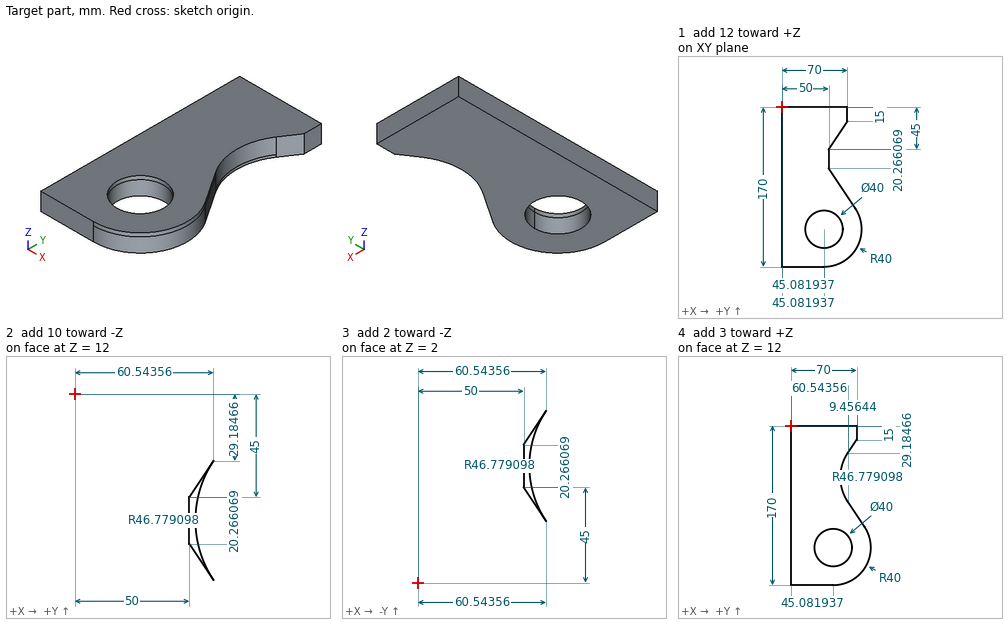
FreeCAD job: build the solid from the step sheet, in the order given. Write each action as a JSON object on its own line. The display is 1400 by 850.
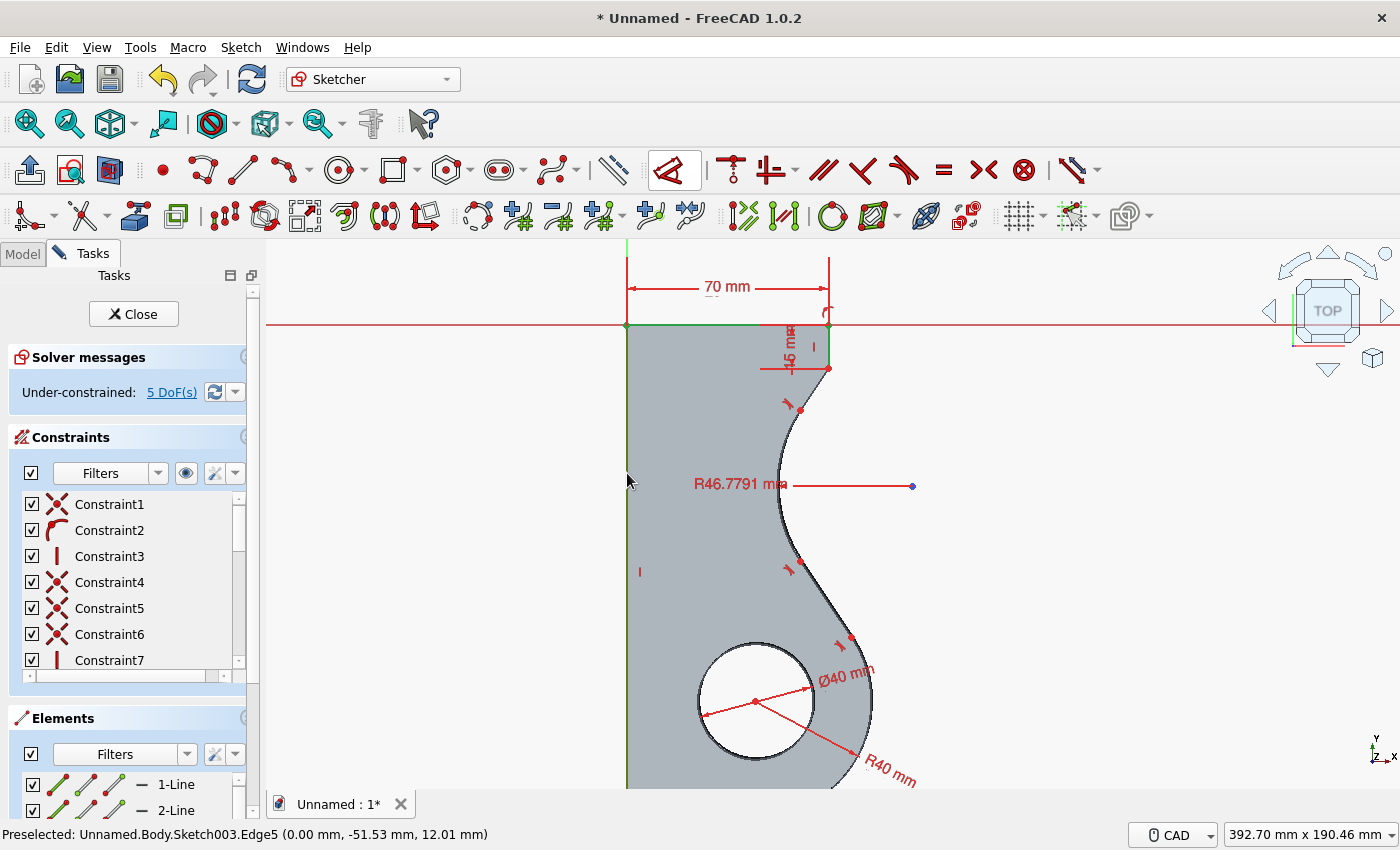
{"action": "key", "text": "i"}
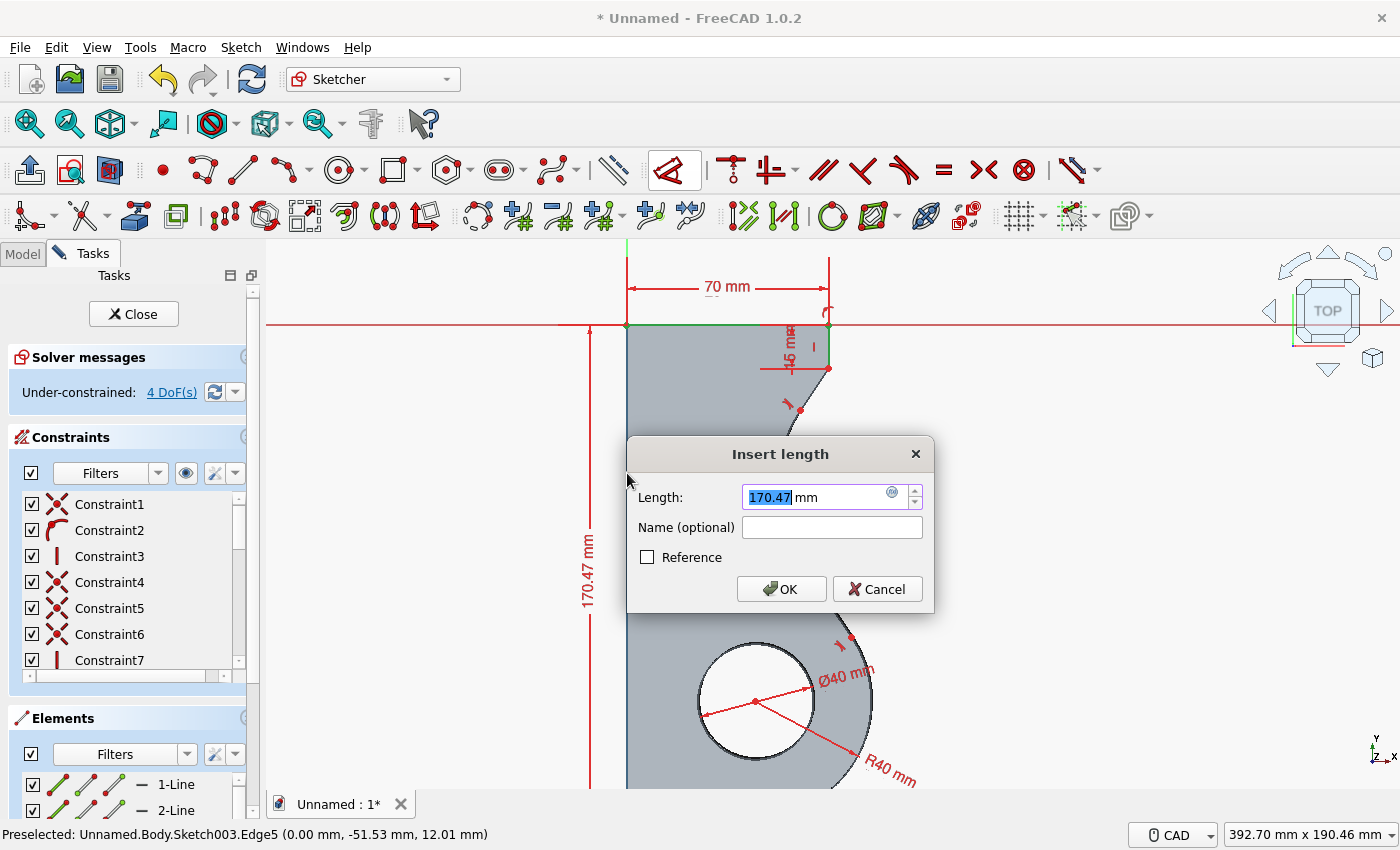
{"action": "type", "text": "170"}
{"action": "key", "text": "Return"}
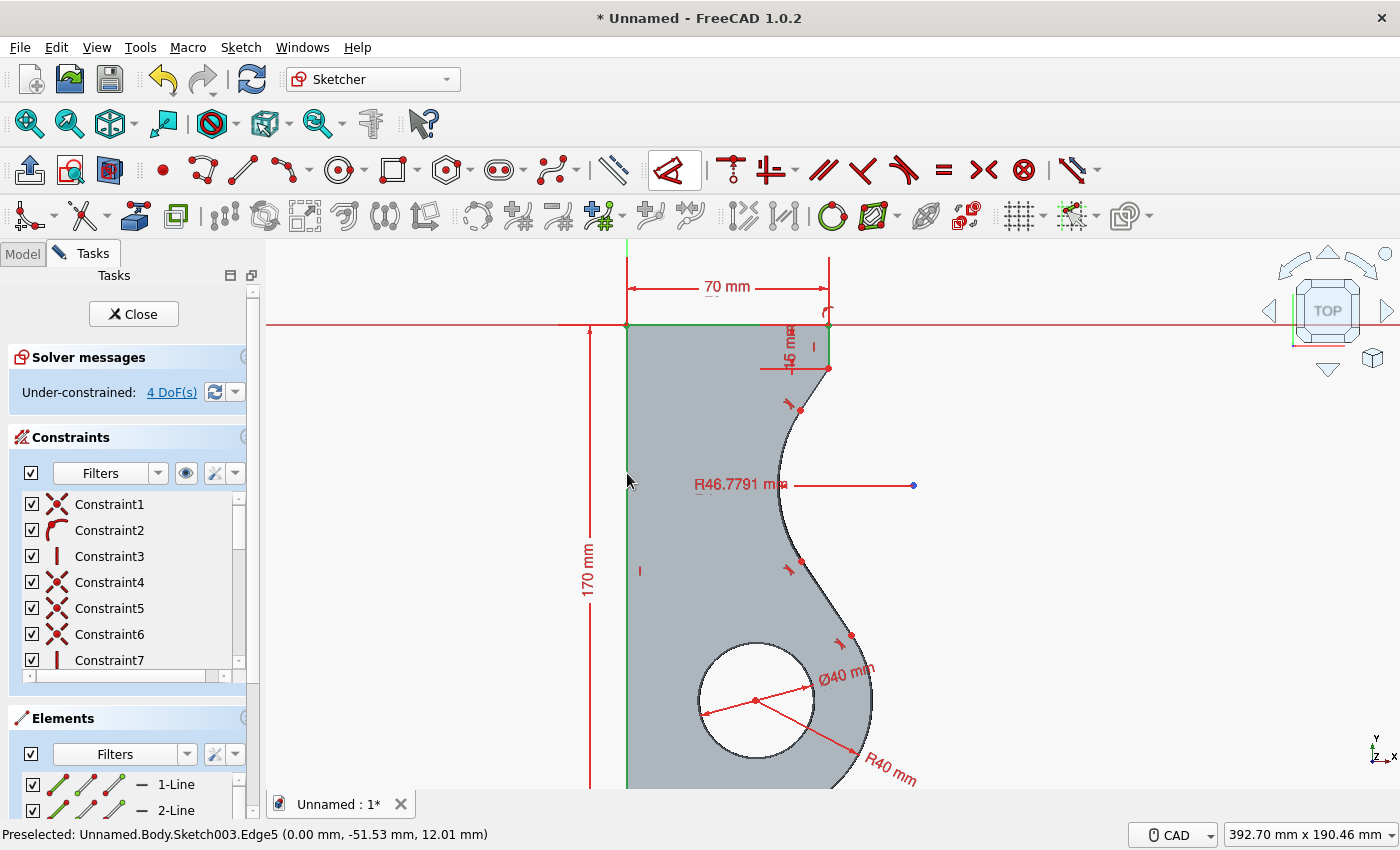
{"action": "scroll", "coordinate": [809, 398], "scroll_direction": "up", "scroll_amount": 2}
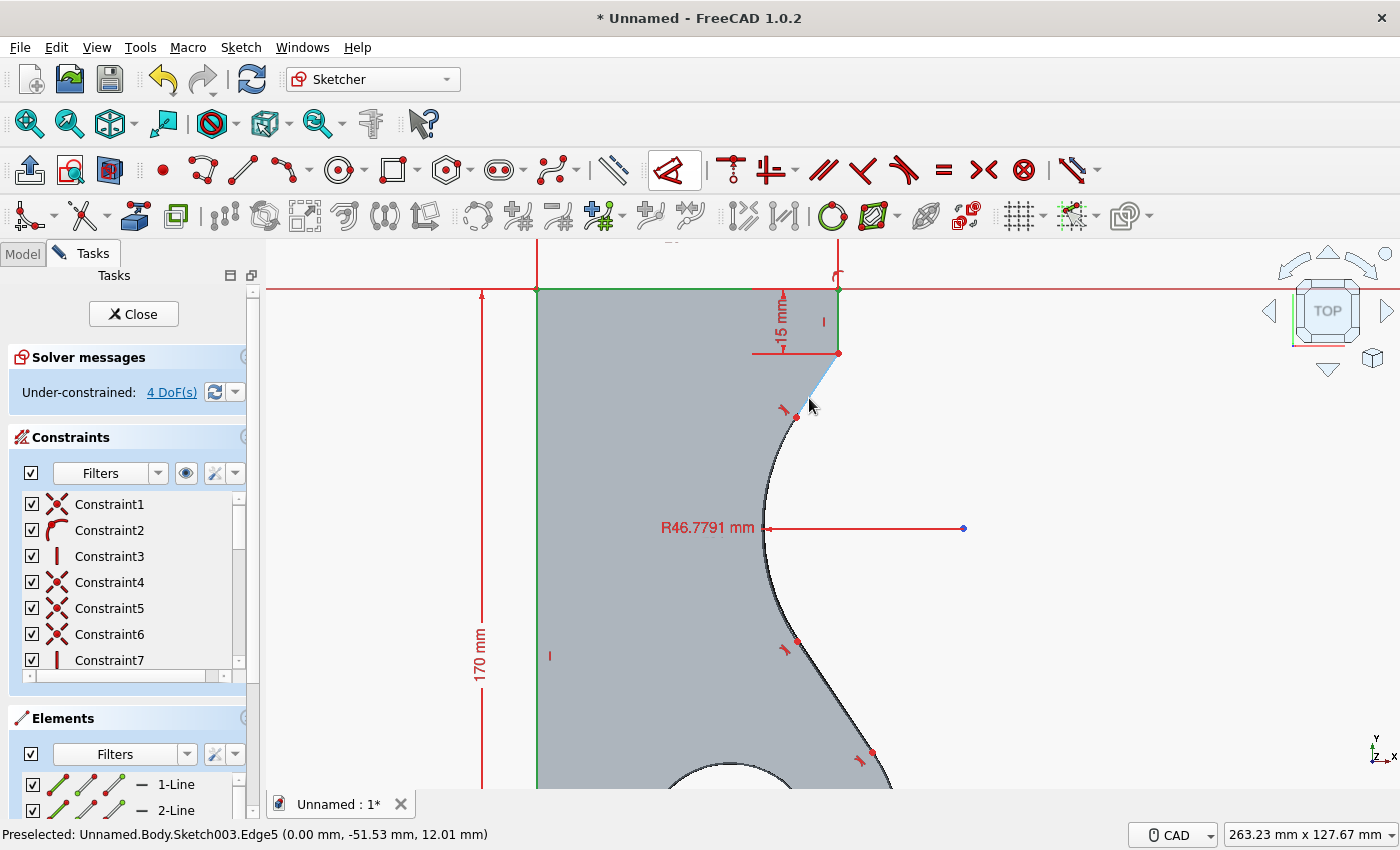
{"action": "left_click", "coordinate": [809, 398]}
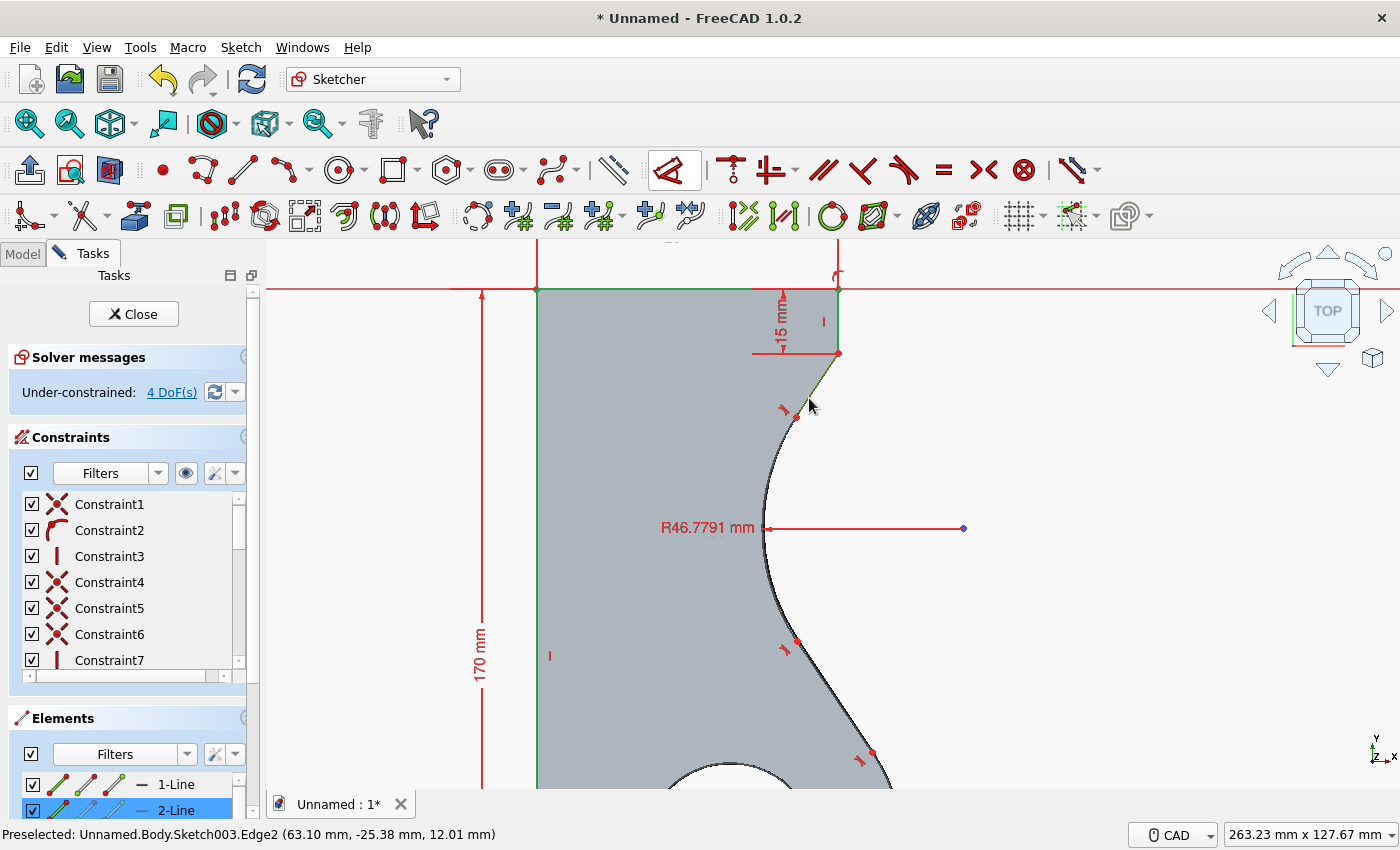
{"action": "key", "text": "l"}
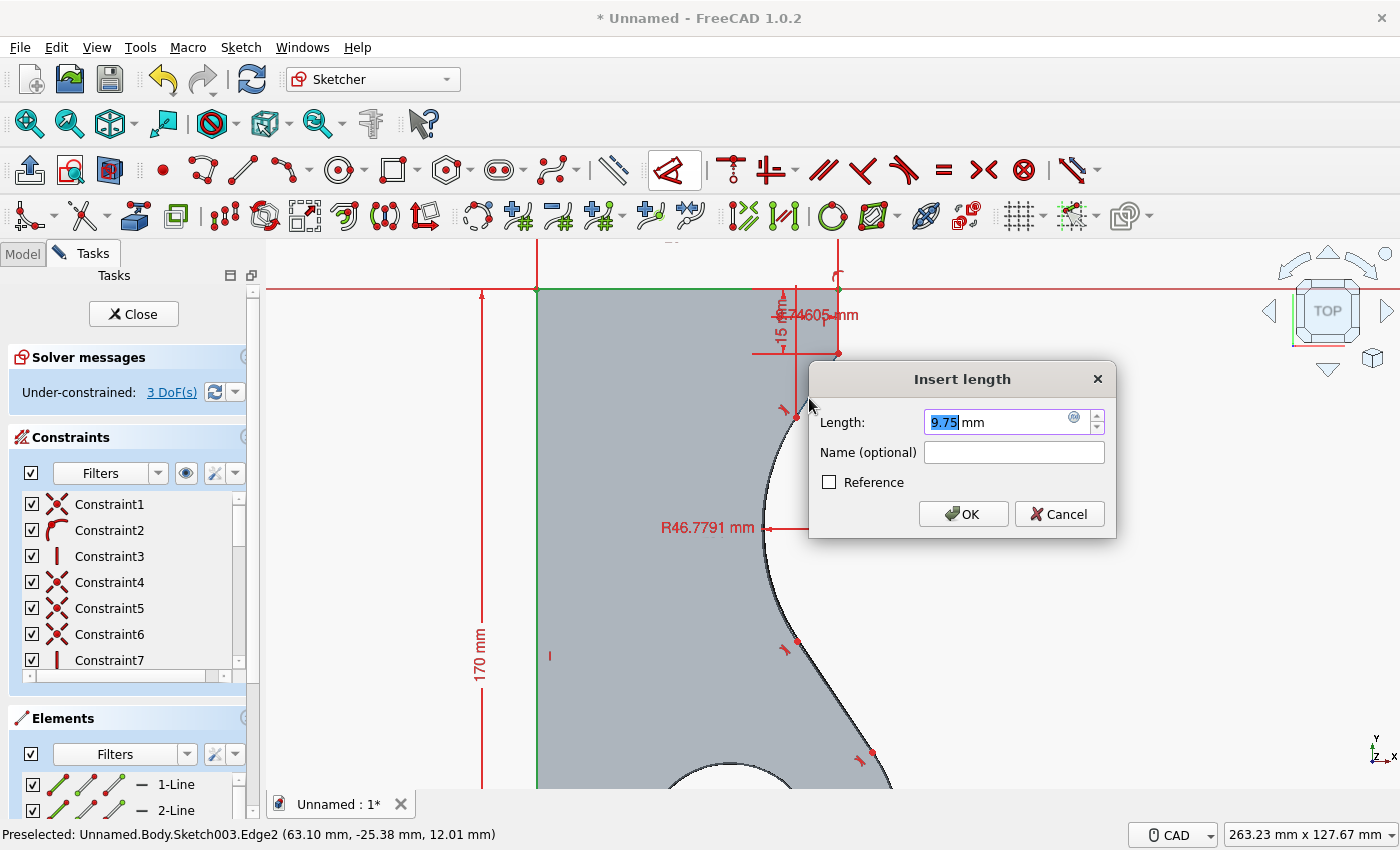
{"action": "type", "text": "9.45644"}
{"action": "key", "text": "Return"}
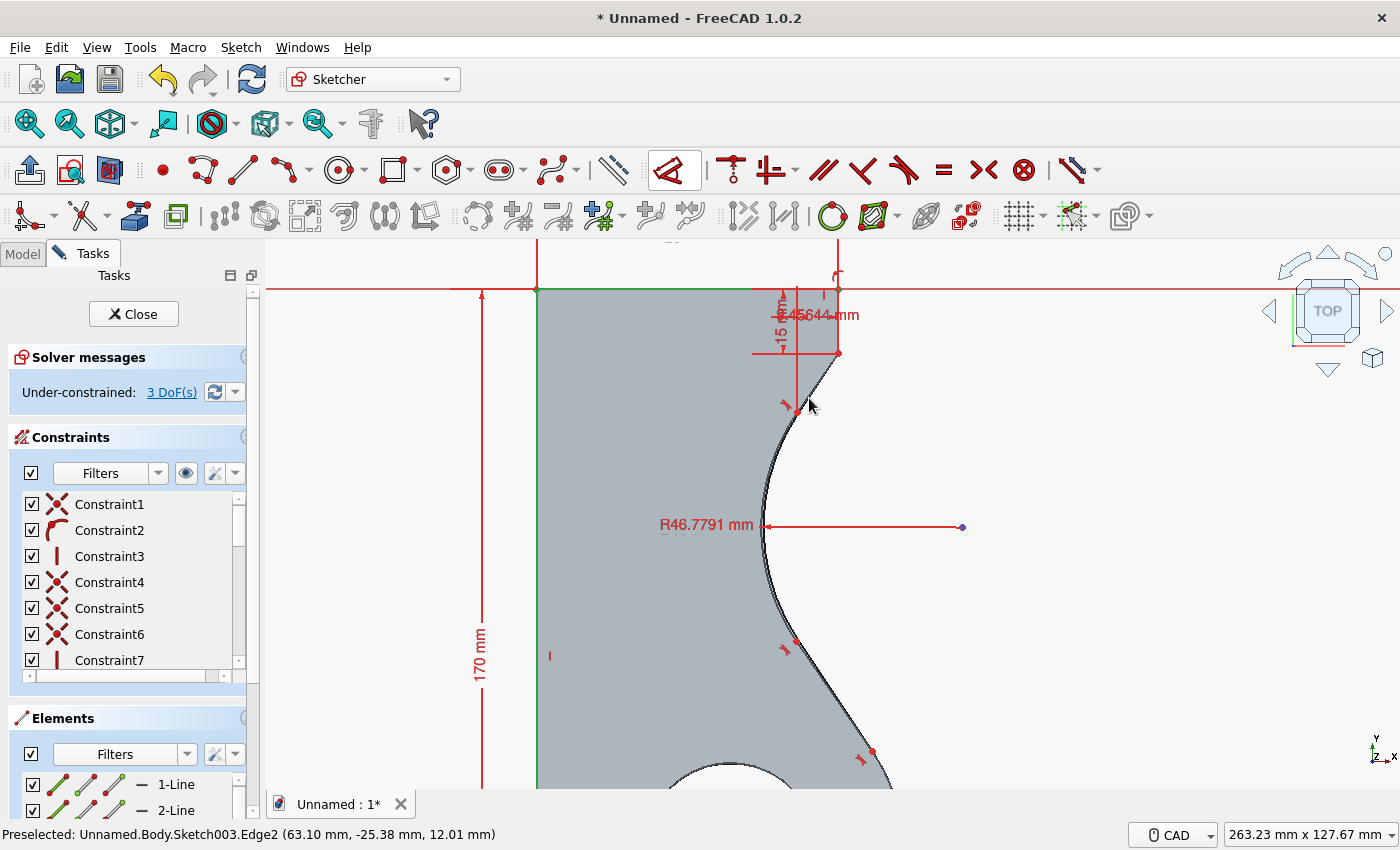
{"action": "scroll", "coordinate": [809, 399], "scroll_direction": "down", "scroll_amount": 4}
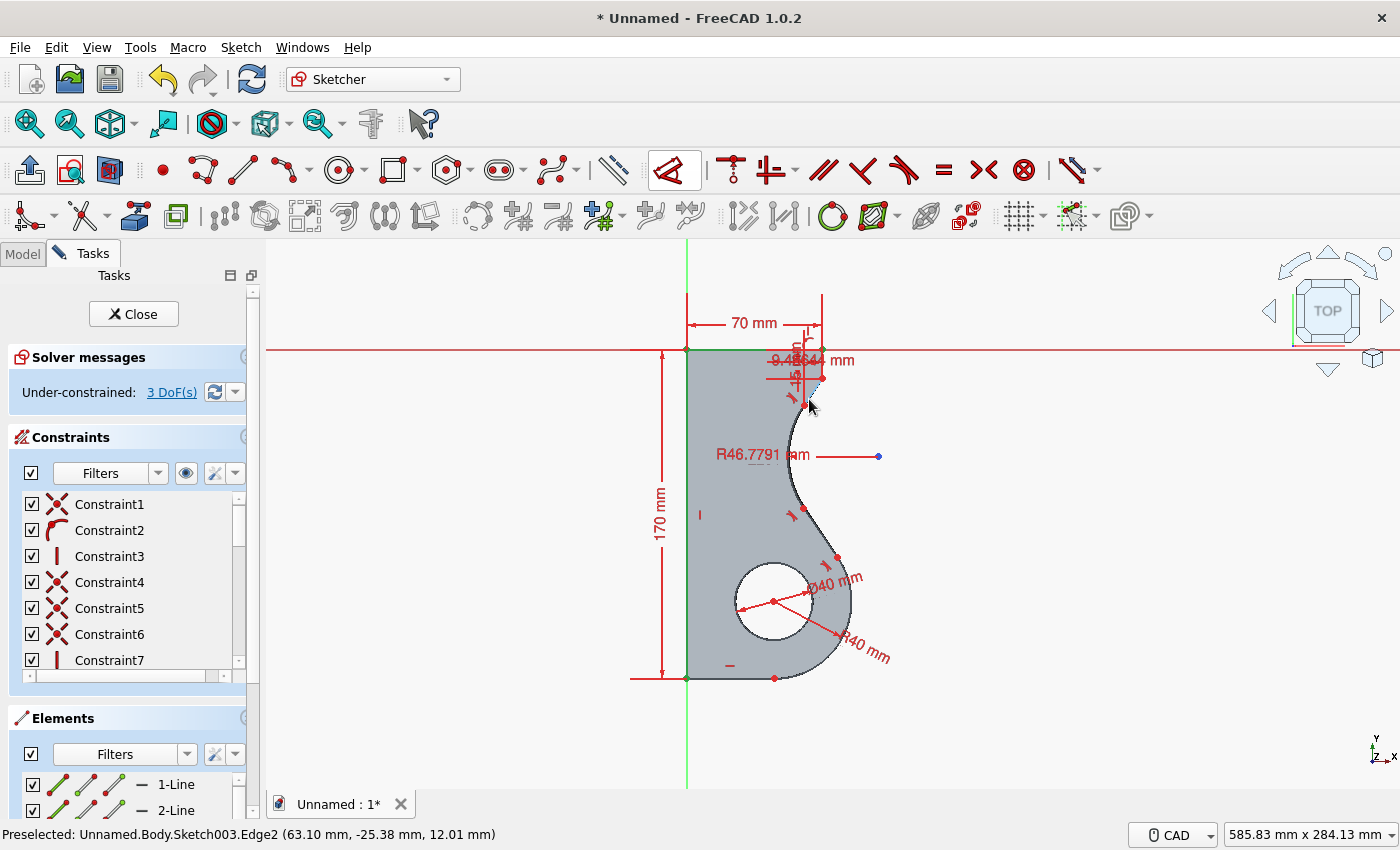
{"action": "left_click", "coordinate": [713, 679]}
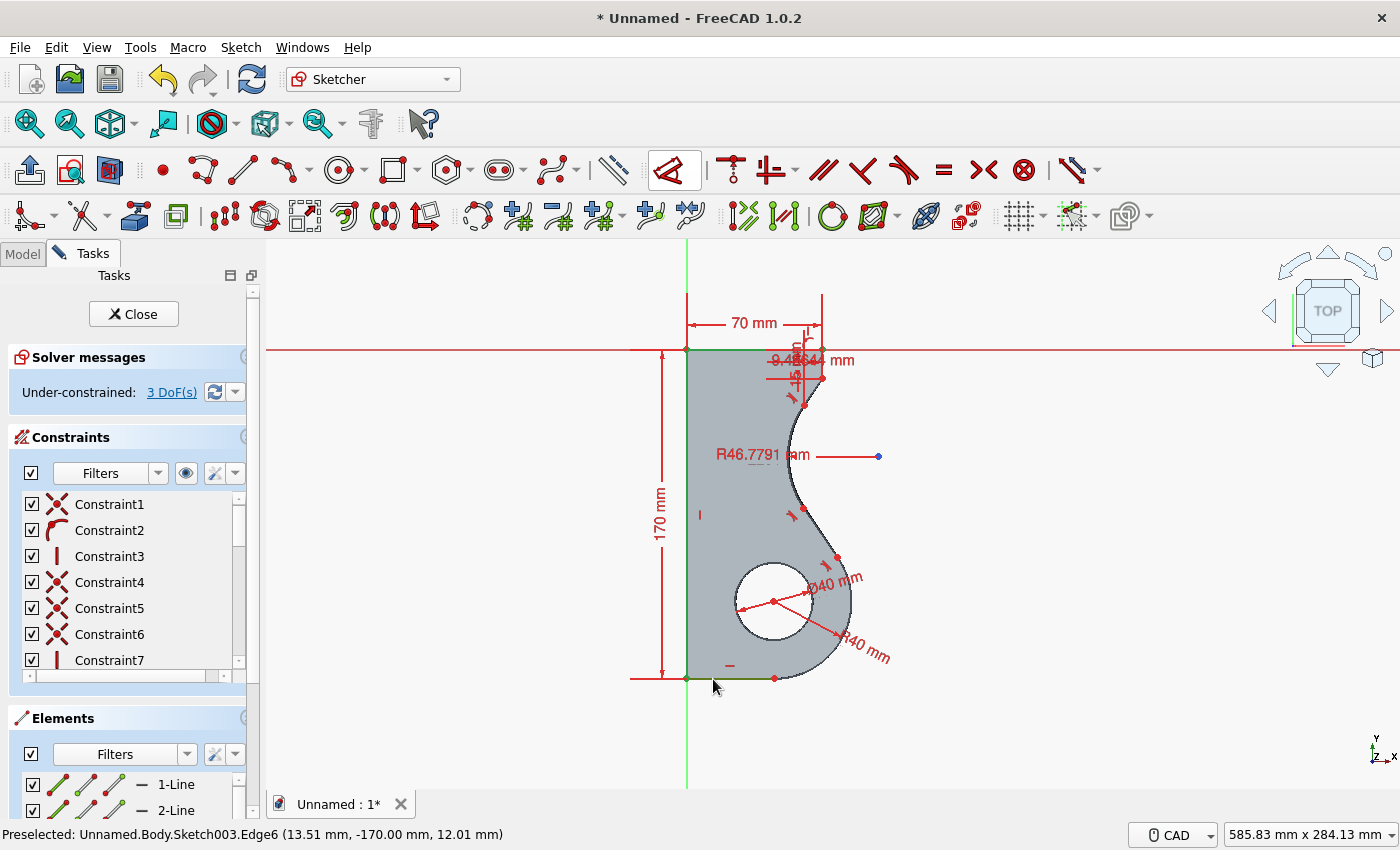
{"action": "left_click", "coordinate": [696, 170]}